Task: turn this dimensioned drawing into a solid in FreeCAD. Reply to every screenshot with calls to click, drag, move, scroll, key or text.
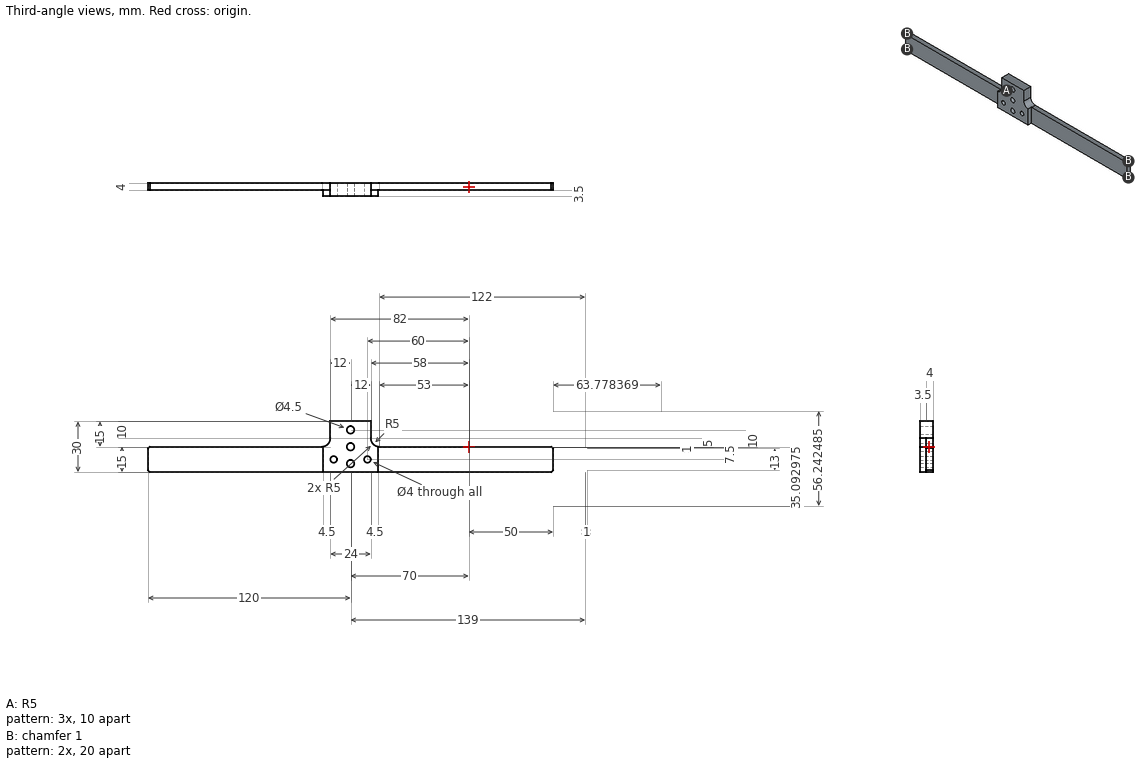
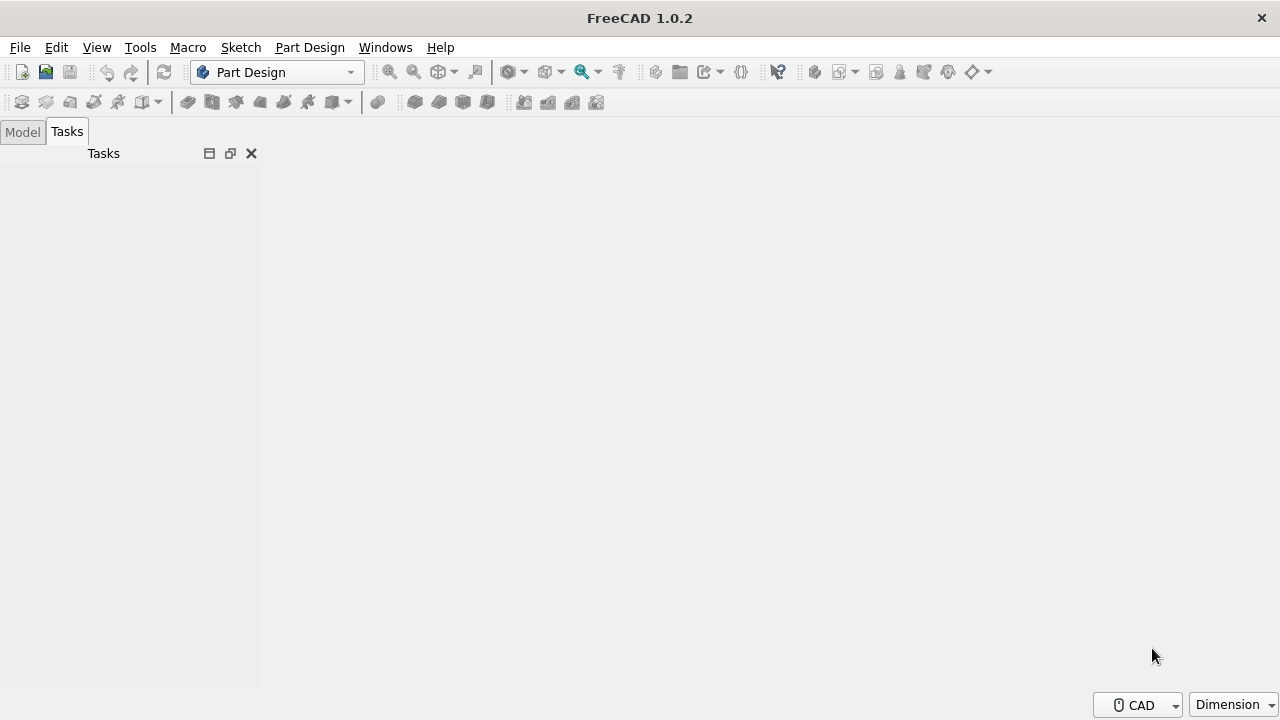
click(22, 72)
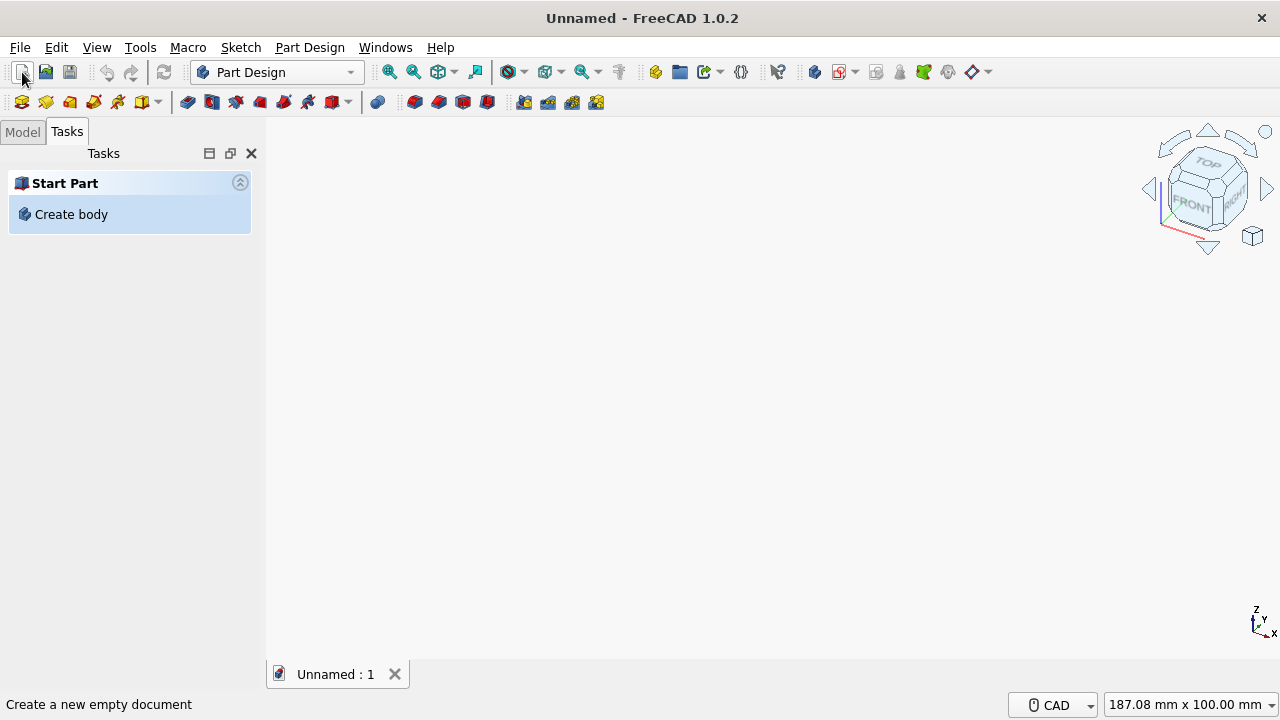
click(816, 72)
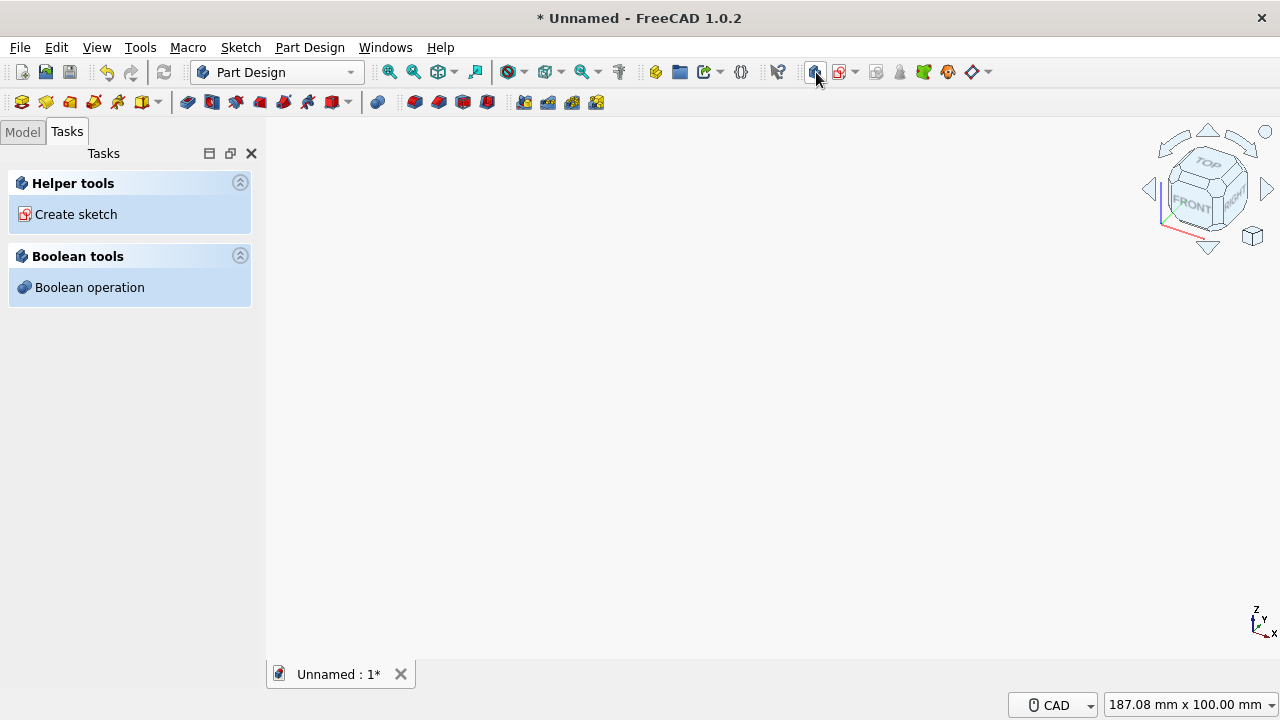
click(23, 131)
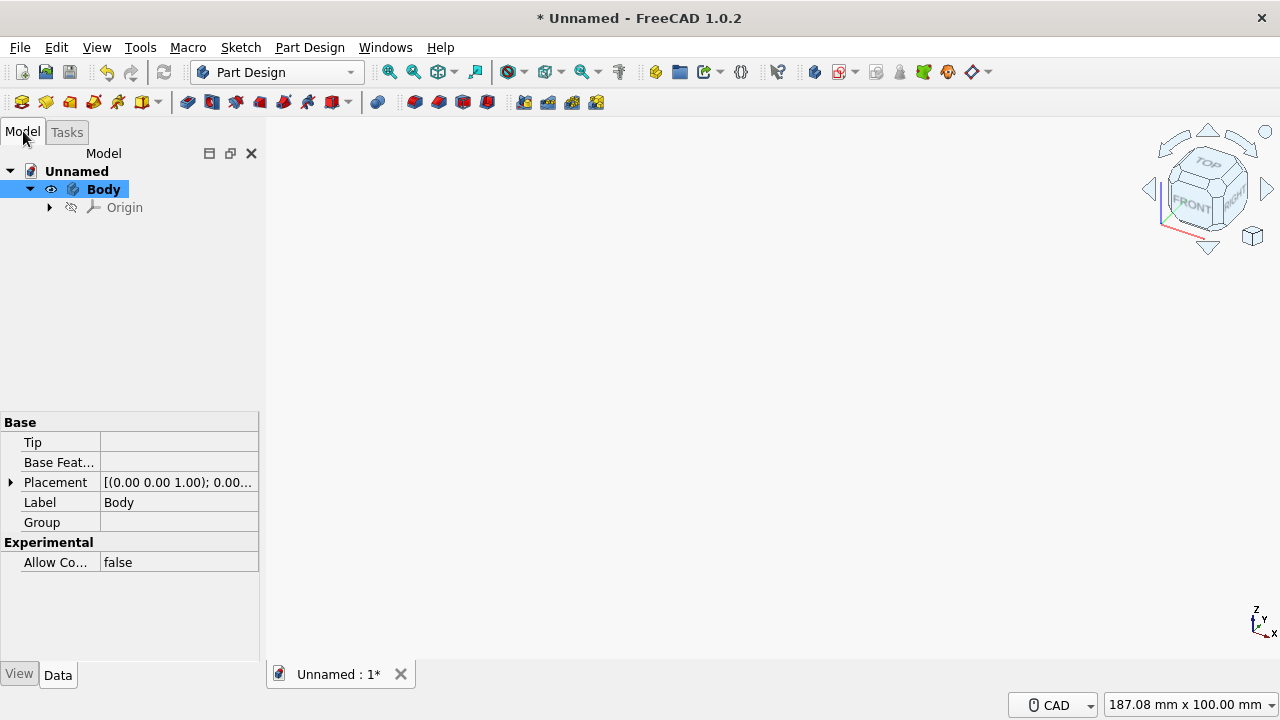
click(50, 207)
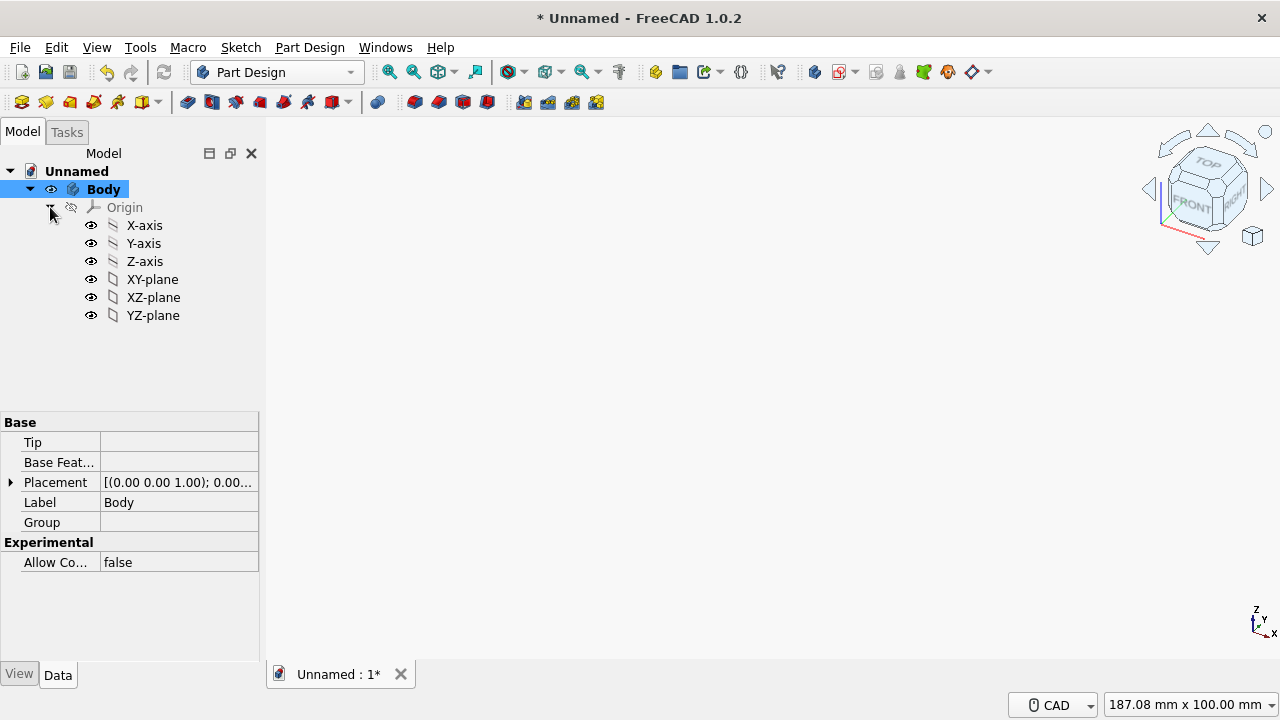
click(136, 297)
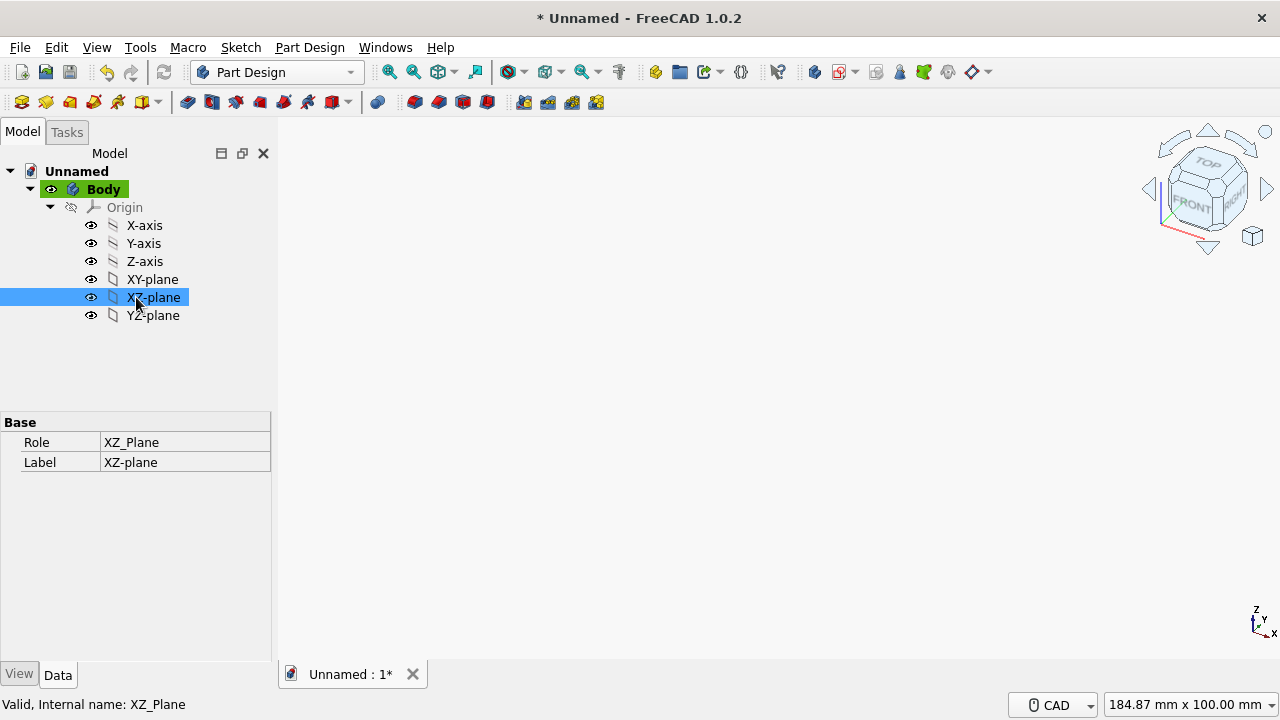
click(972, 72)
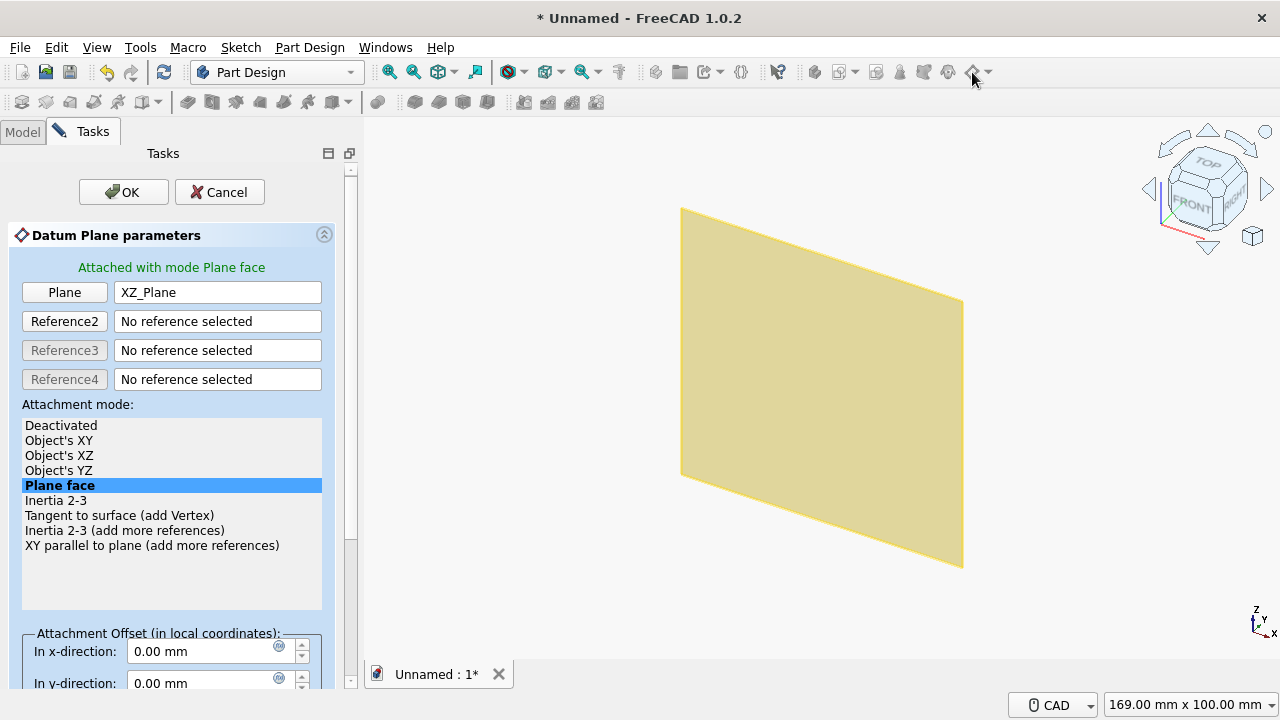
scroll(351, 426, down, 2)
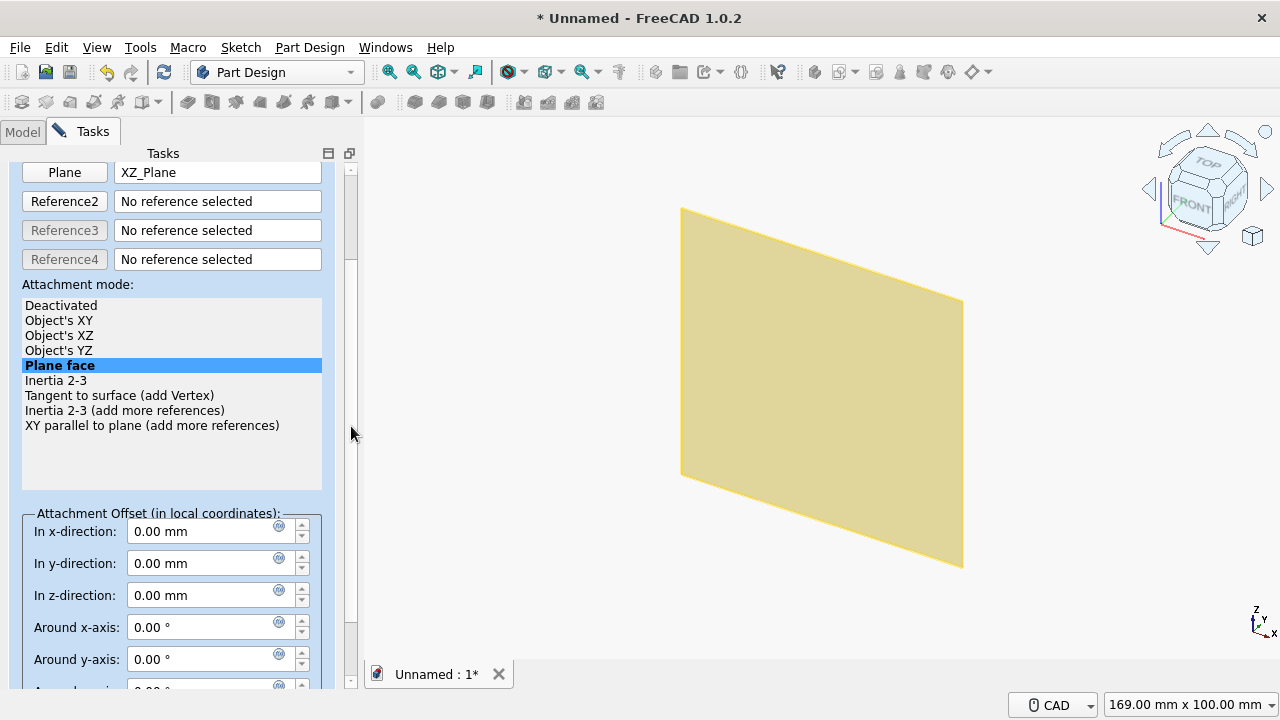
triple_click(210, 595)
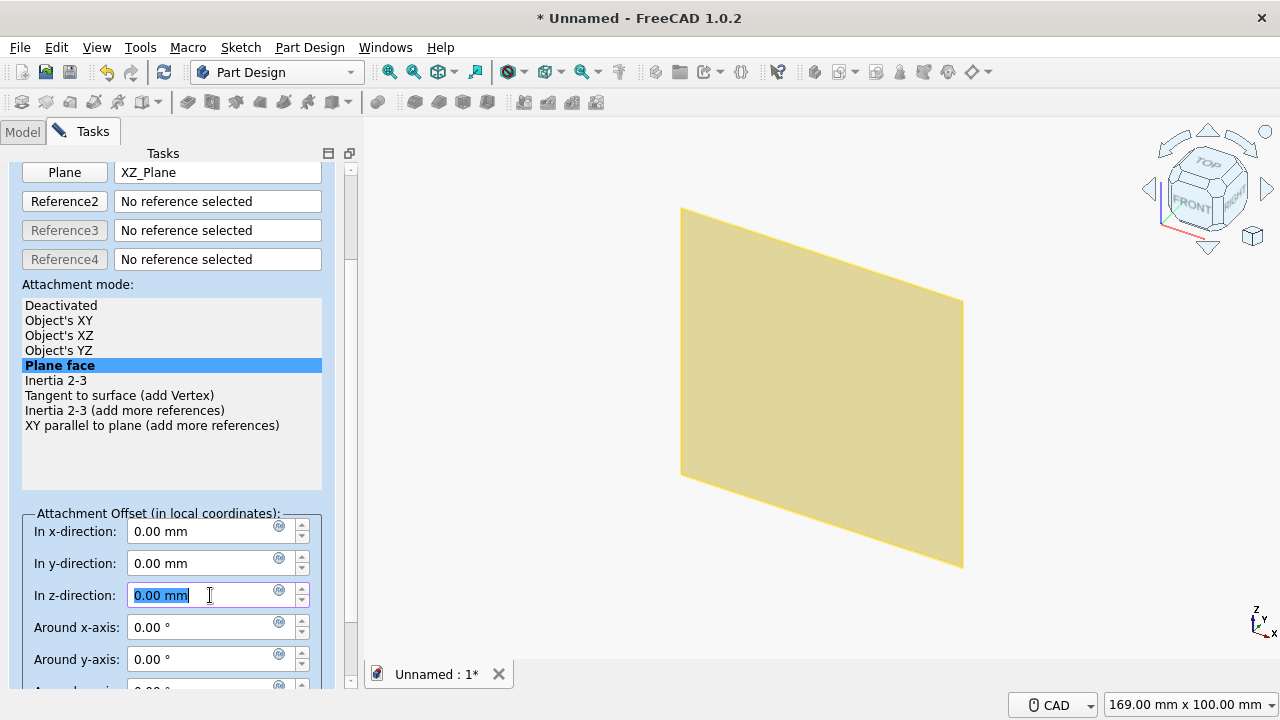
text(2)
key(Tab)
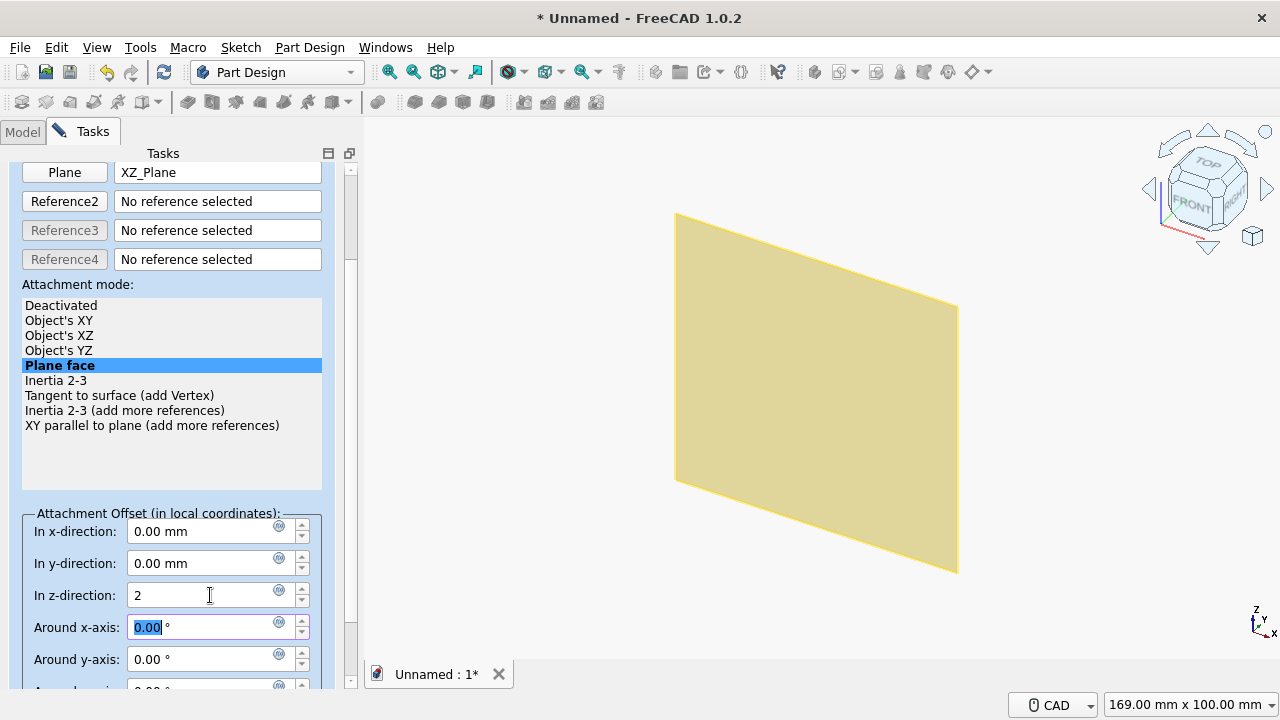
scroll(351, 426, up, 3)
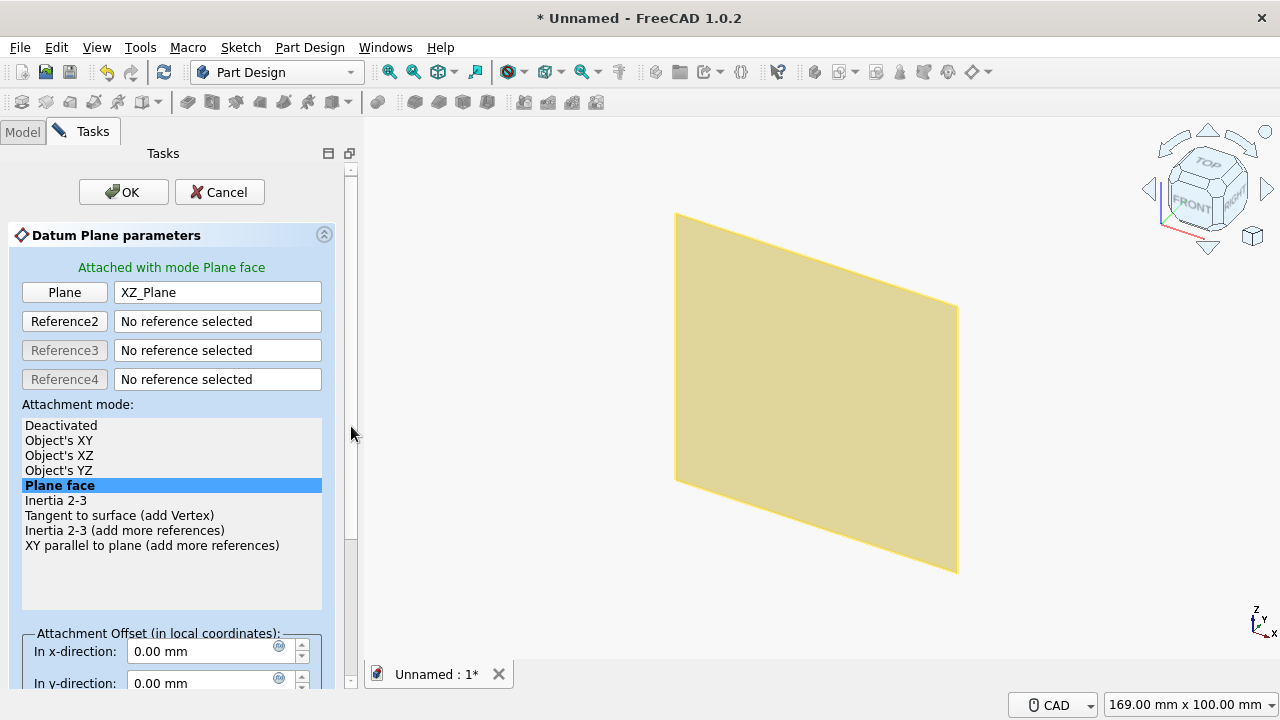
click(124, 192)